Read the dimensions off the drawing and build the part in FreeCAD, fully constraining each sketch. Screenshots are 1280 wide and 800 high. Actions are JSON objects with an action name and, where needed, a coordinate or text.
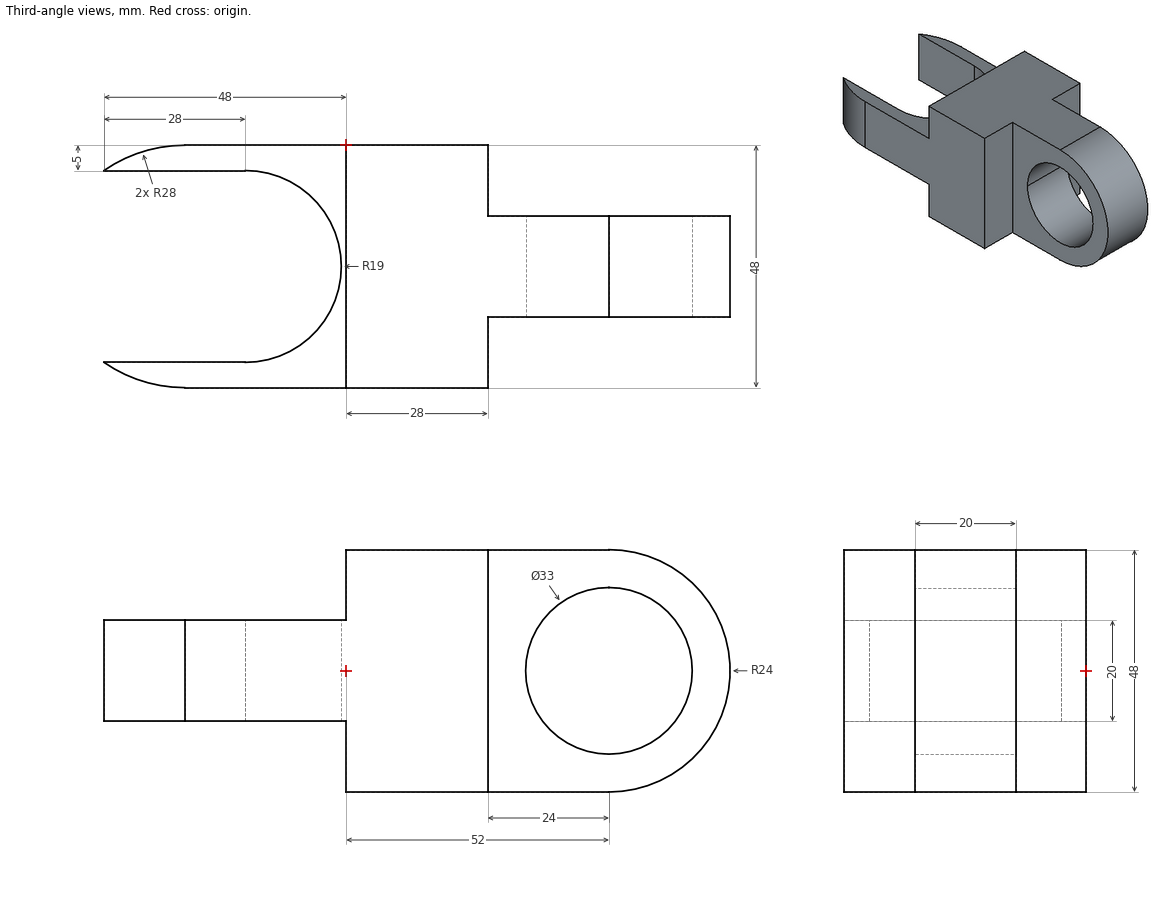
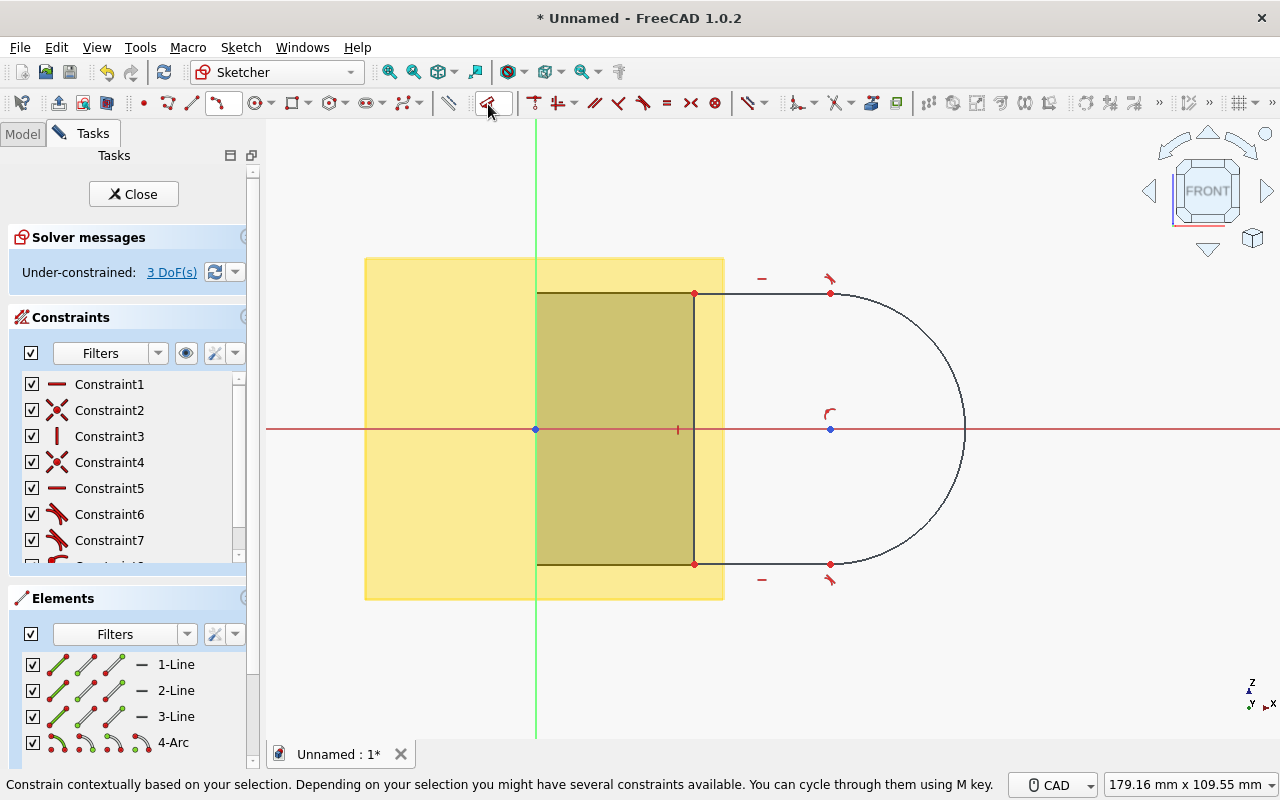
{"action": "left_click", "coordinate": [939, 509]}
{"action": "left_click", "coordinate": [965, 528]}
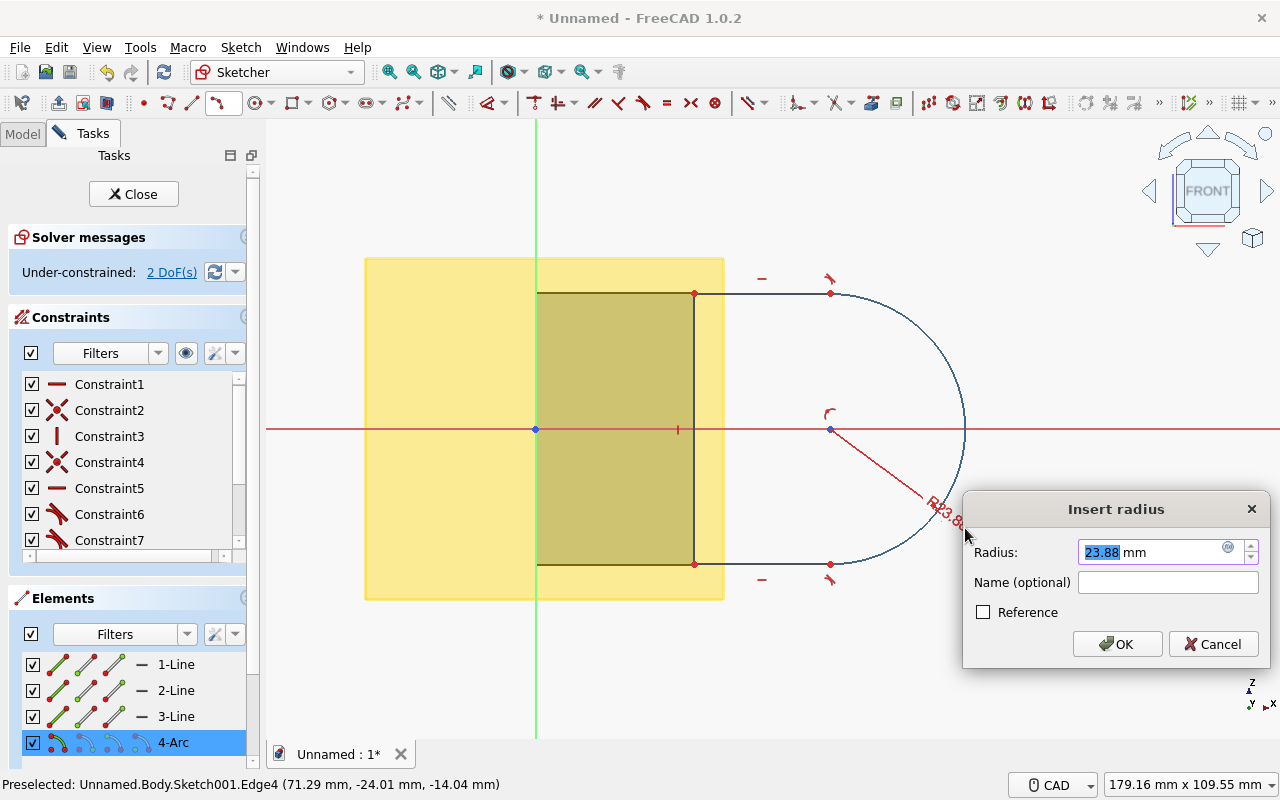
{"action": "type", "text": "24"}
{"action": "key", "text": "Return"}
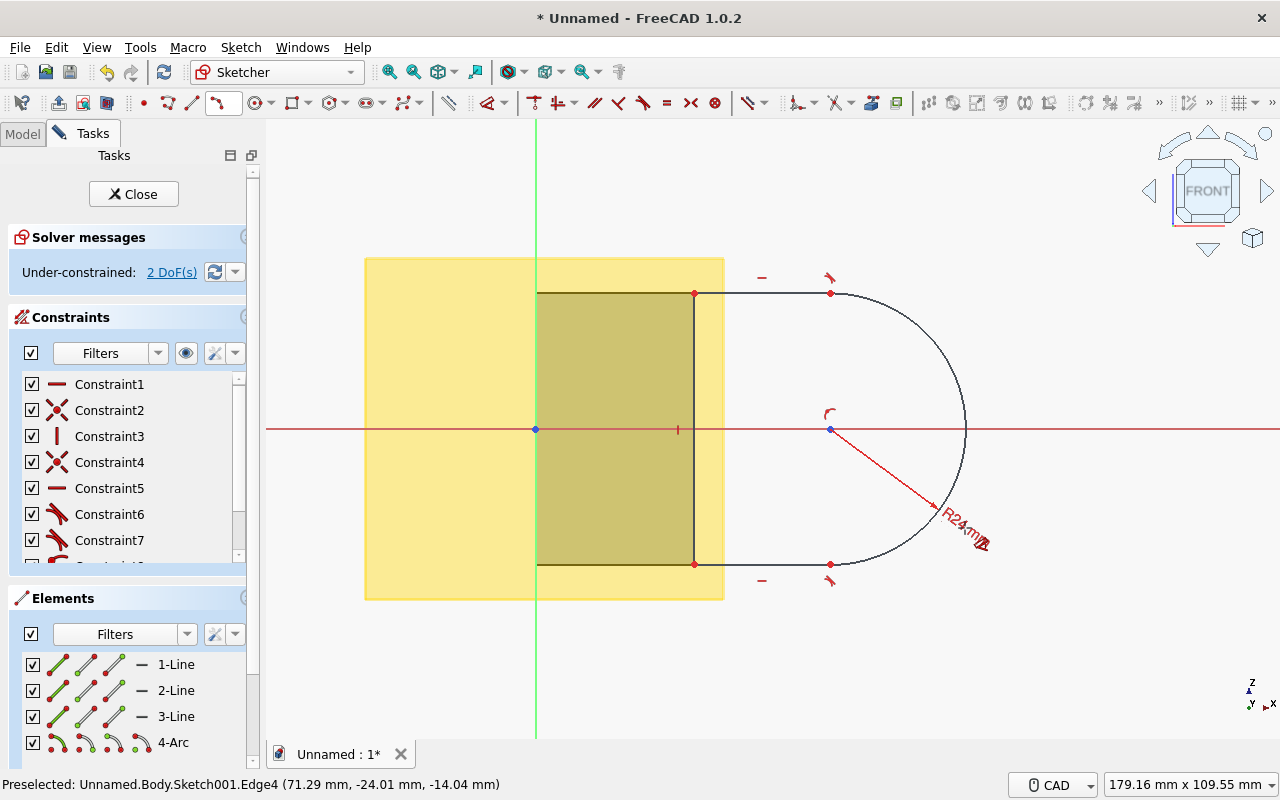
{"action": "left_click", "coordinate": [789, 565]}
{"action": "left_click", "coordinate": [762, 599]}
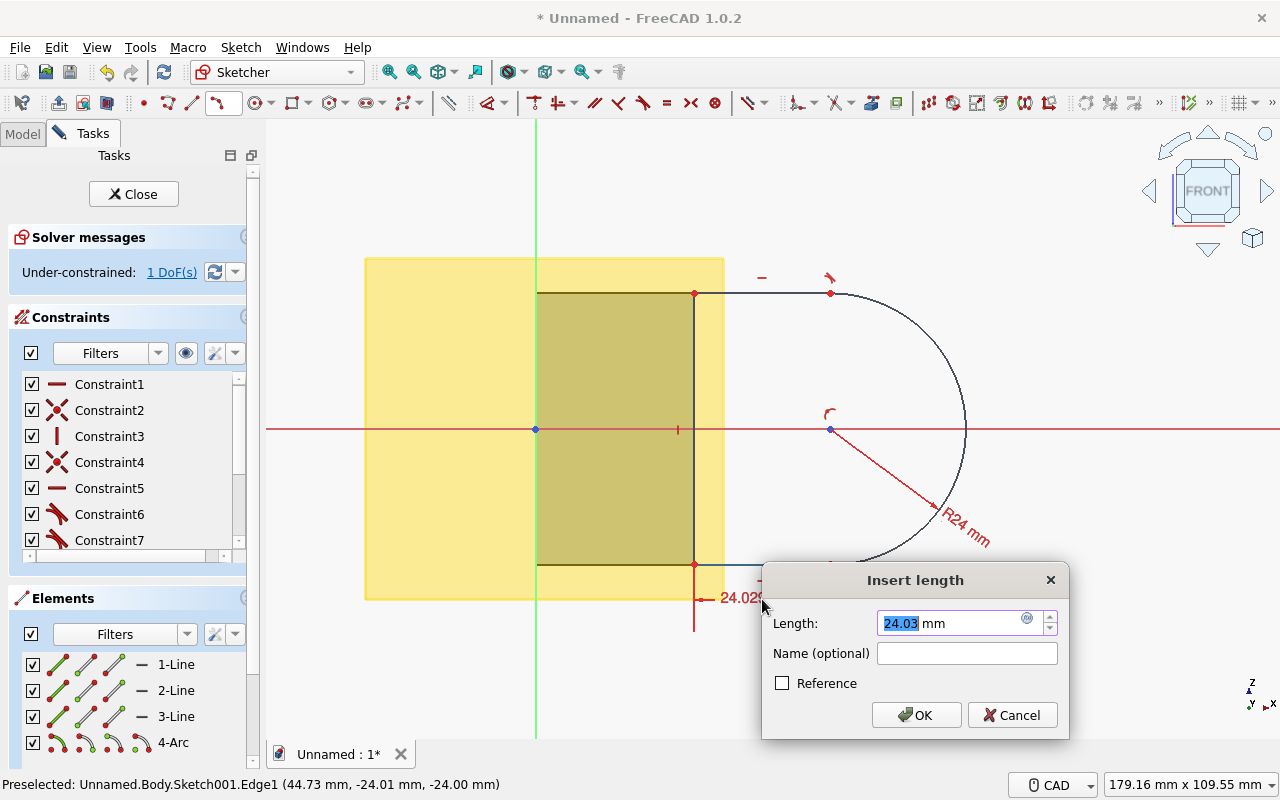
{"action": "type", "text": "24"}
{"action": "key", "text": "Return"}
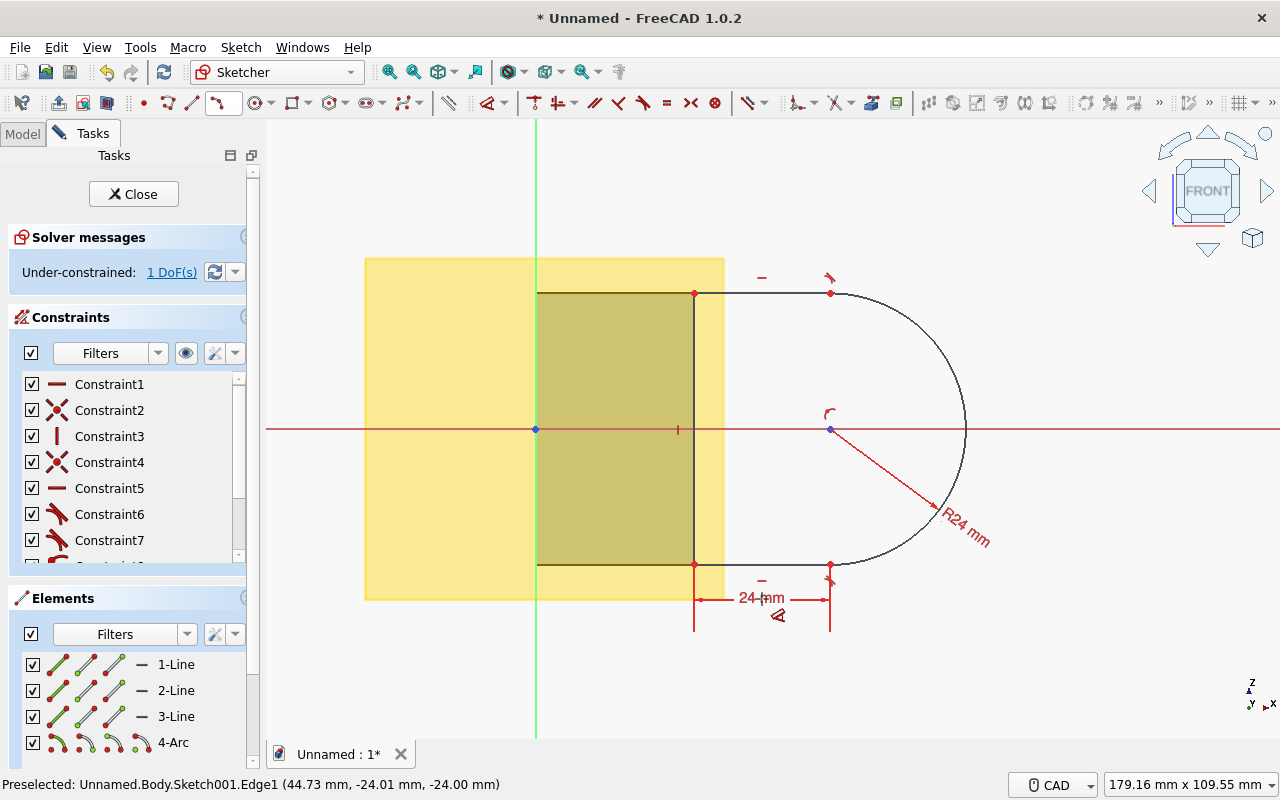
{"action": "left_click", "coordinate": [830, 565]}
{"action": "left_click", "coordinate": [683, 599]}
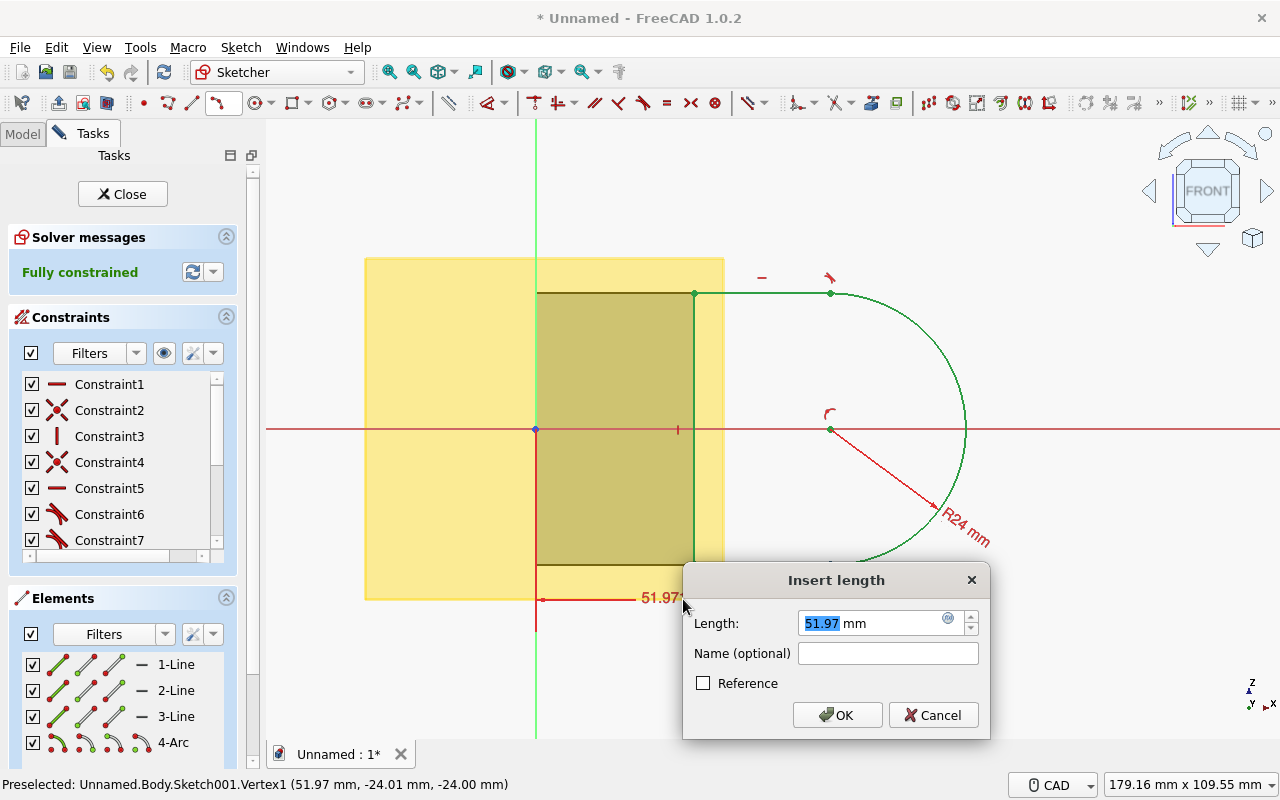
{"action": "type", "text": "52"}
{"action": "key", "text": "Return"}
{"action": "key", "text": "Escape"}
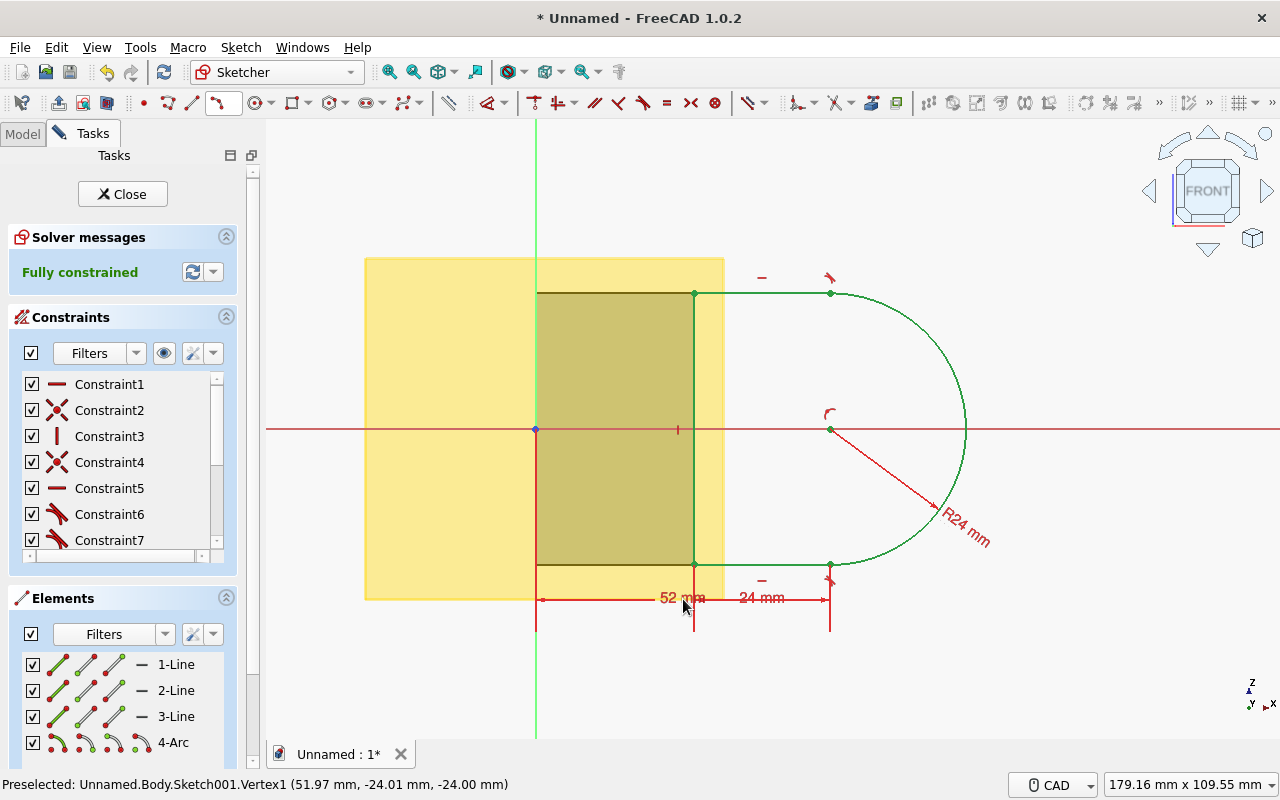
{"action": "left_click", "coordinate": [123, 194]}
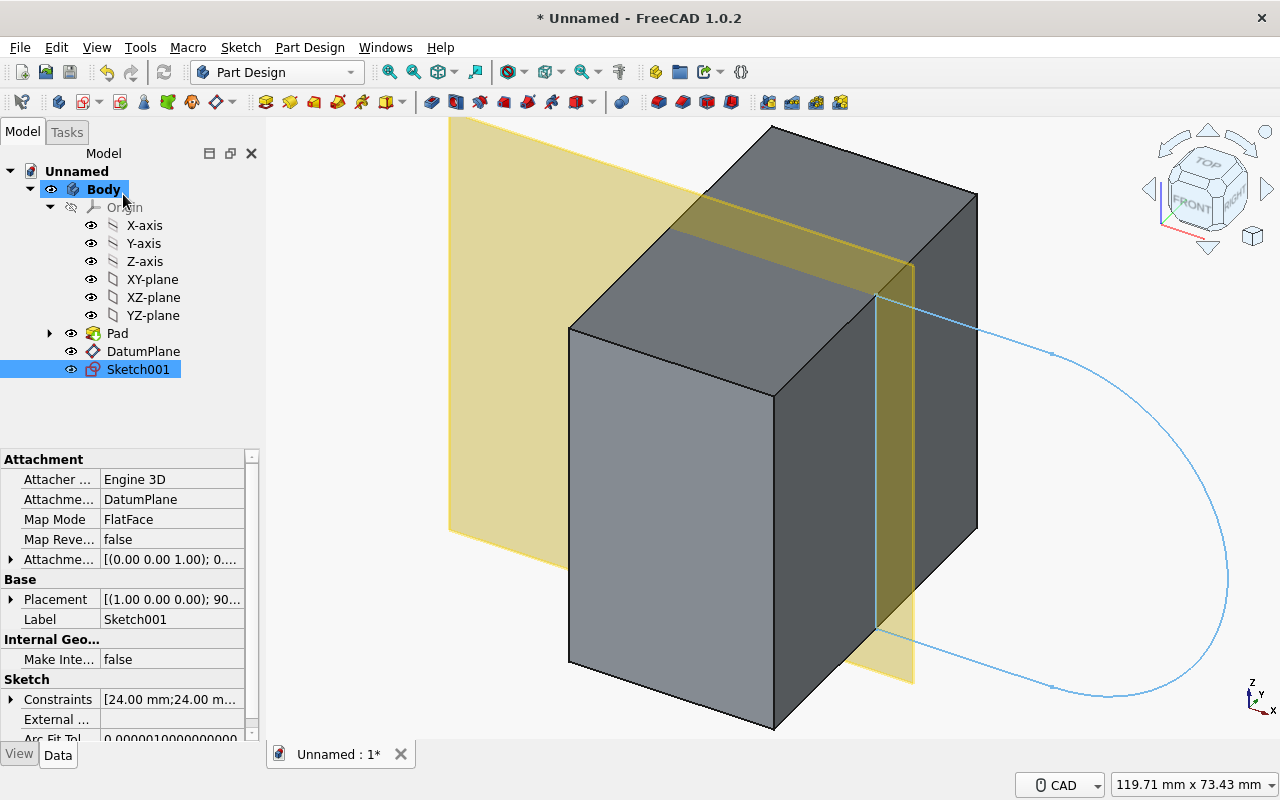
{"action": "left_click", "coordinate": [266, 102]}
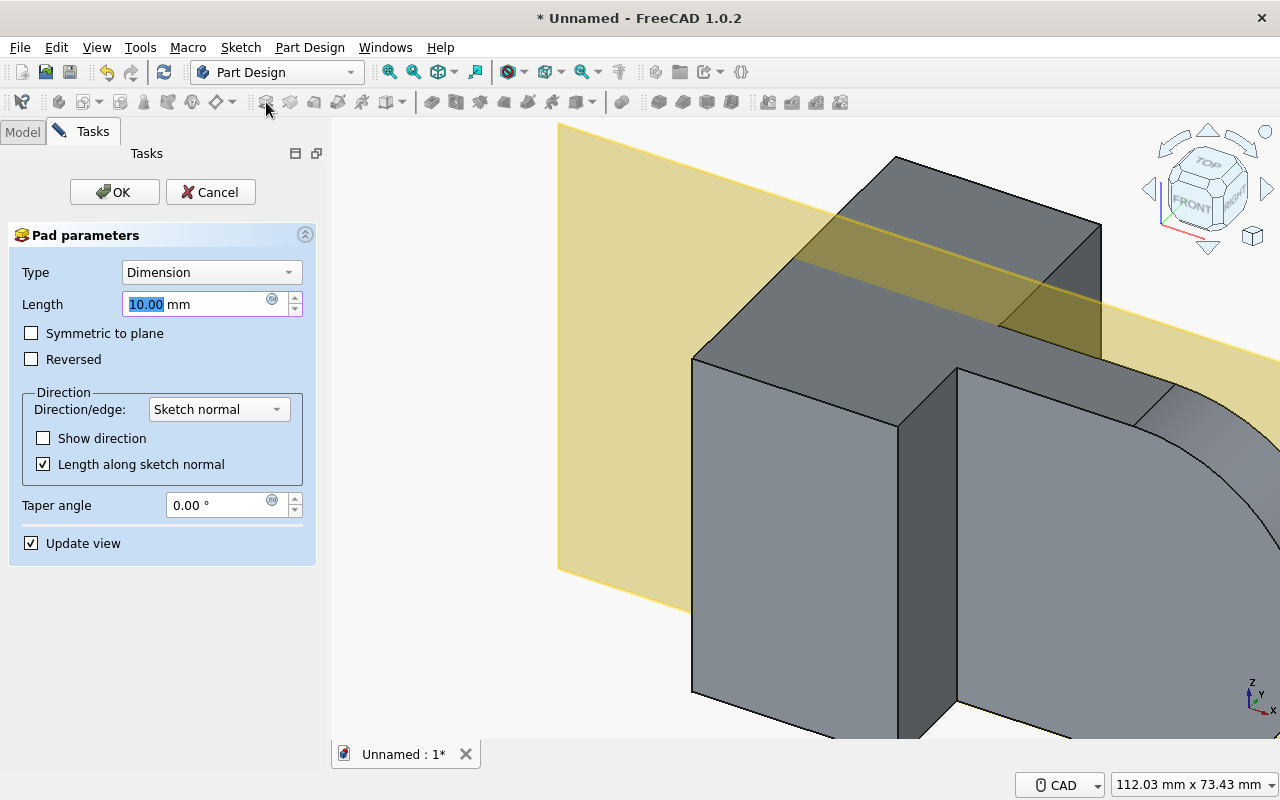
{"action": "type", "text": "20"}
{"action": "key", "text": "Tab"}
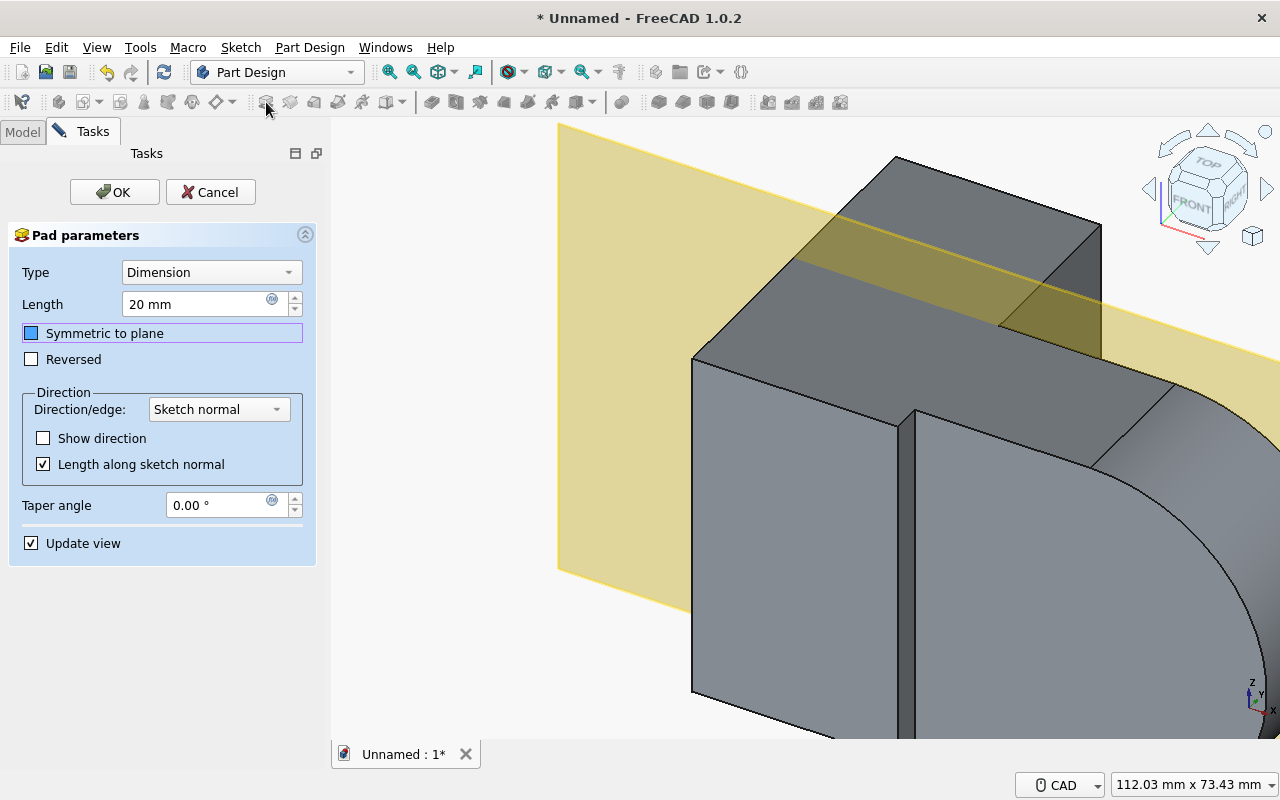
{"action": "left_click", "coordinate": [30, 333]}